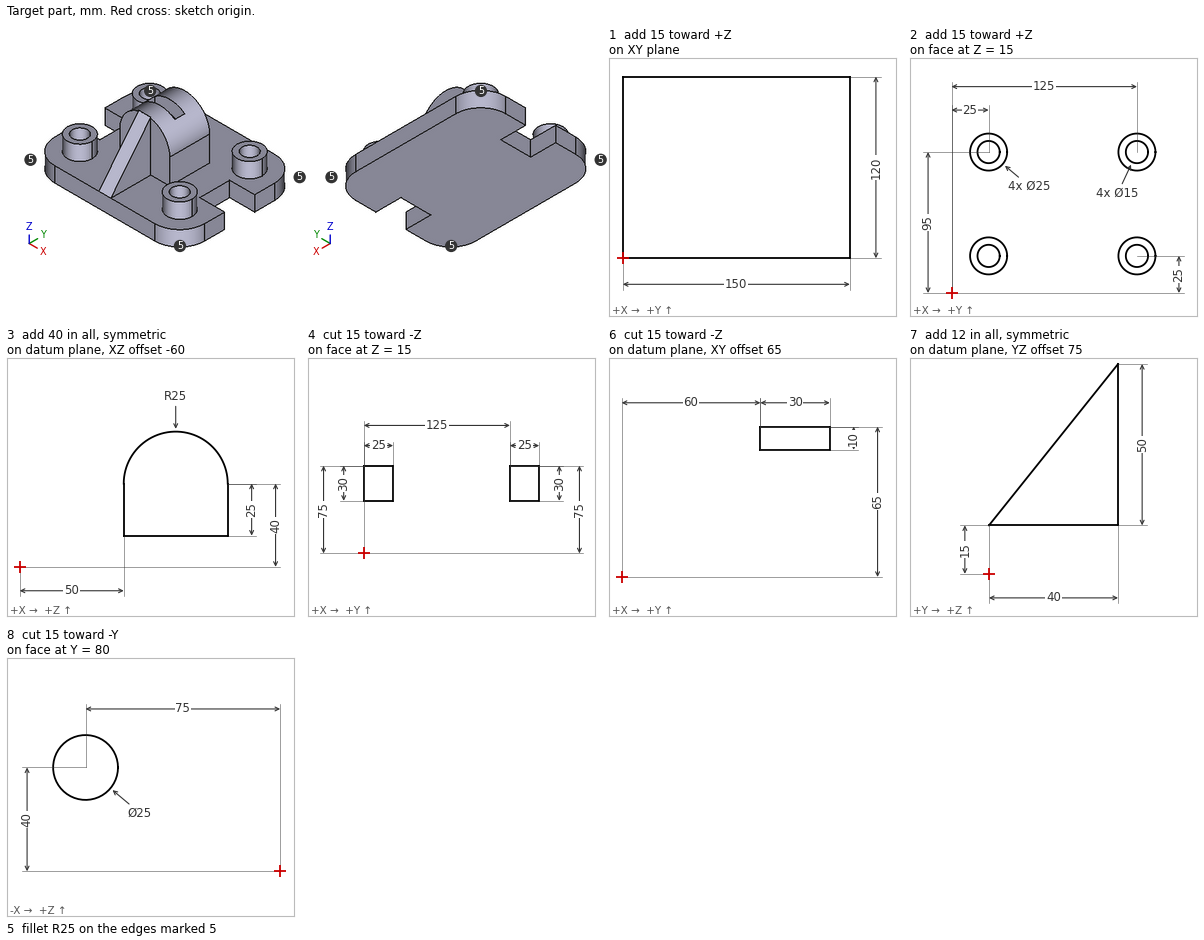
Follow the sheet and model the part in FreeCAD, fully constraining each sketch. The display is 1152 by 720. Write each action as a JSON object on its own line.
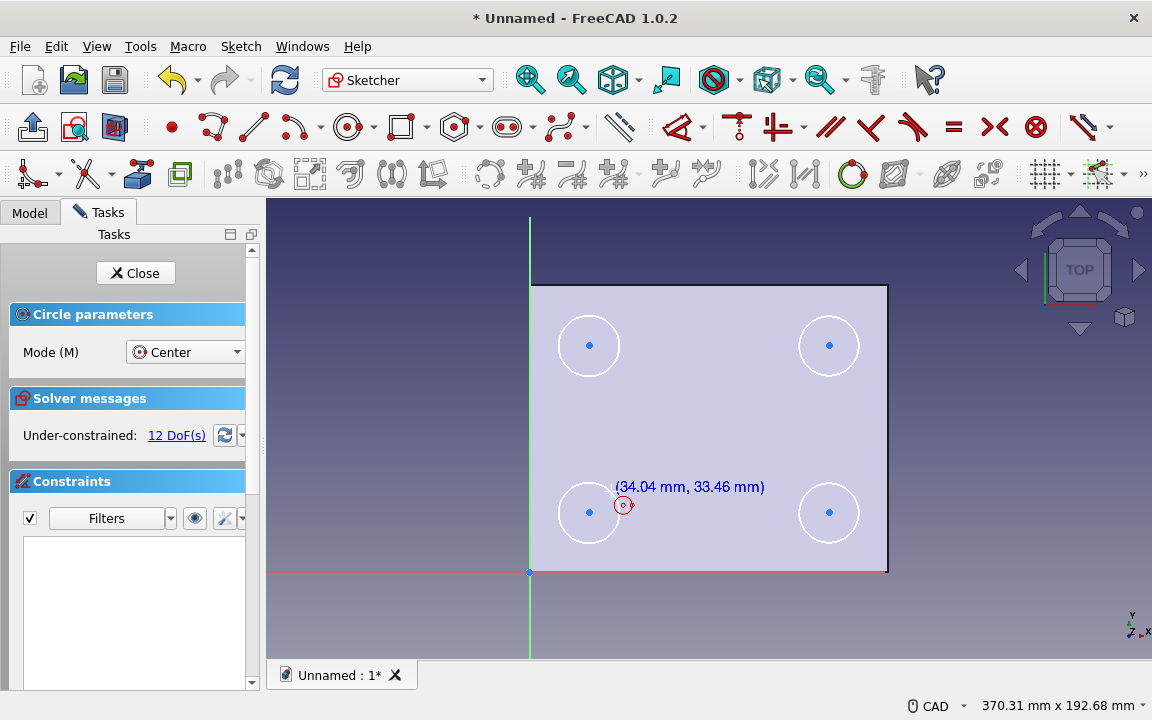
{"action": "scroll", "coordinate": [589, 345], "scroll_direction": "up", "scroll_amount": 2}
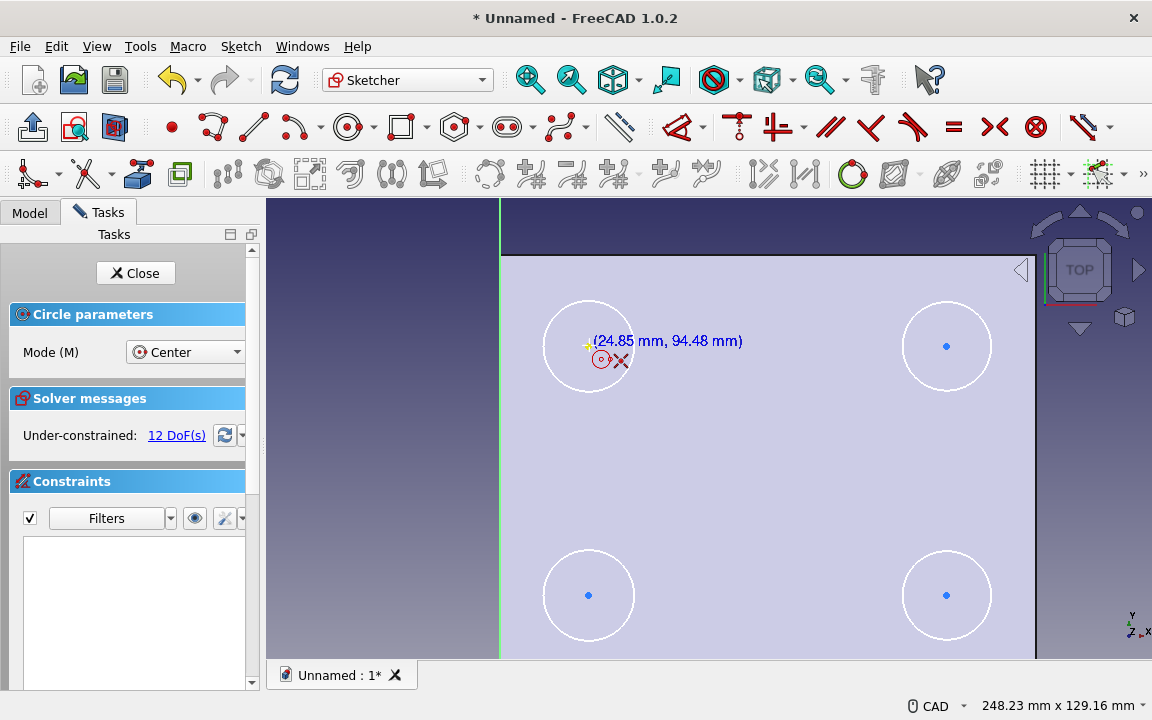
{"action": "left_click", "coordinate": [589, 346]}
{"action": "left_click", "coordinate": [608, 326]}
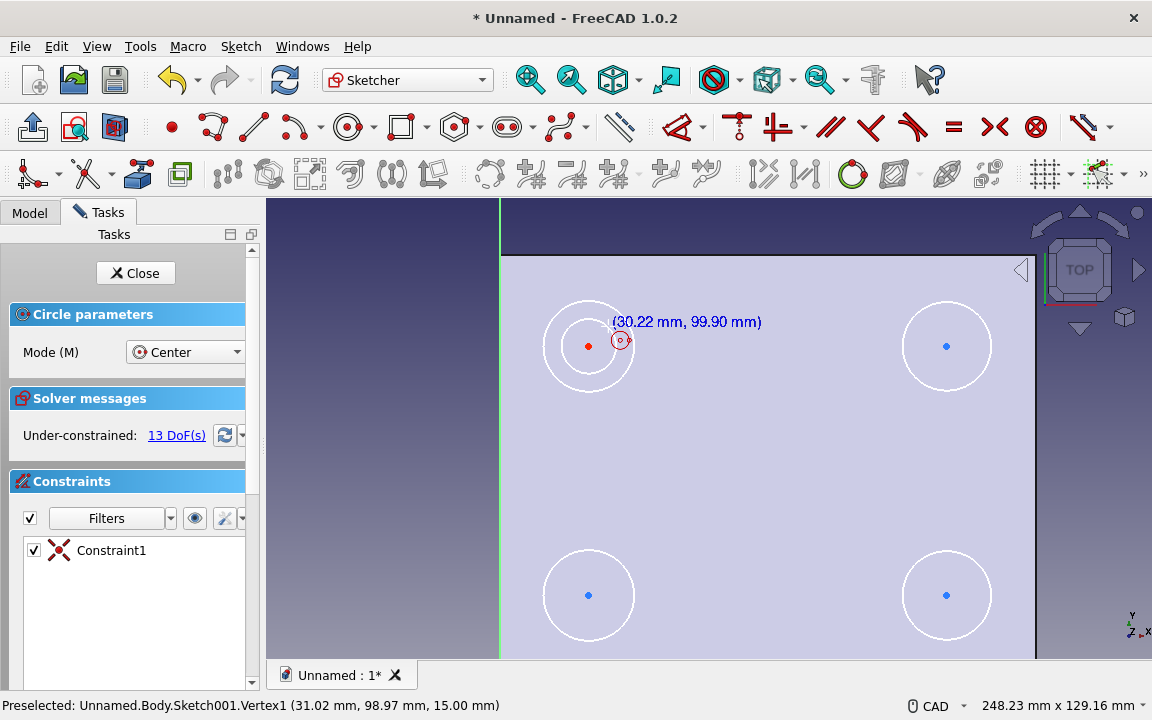
{"action": "left_click", "coordinate": [947, 346]}
{"action": "left_click", "coordinate": [965, 326]}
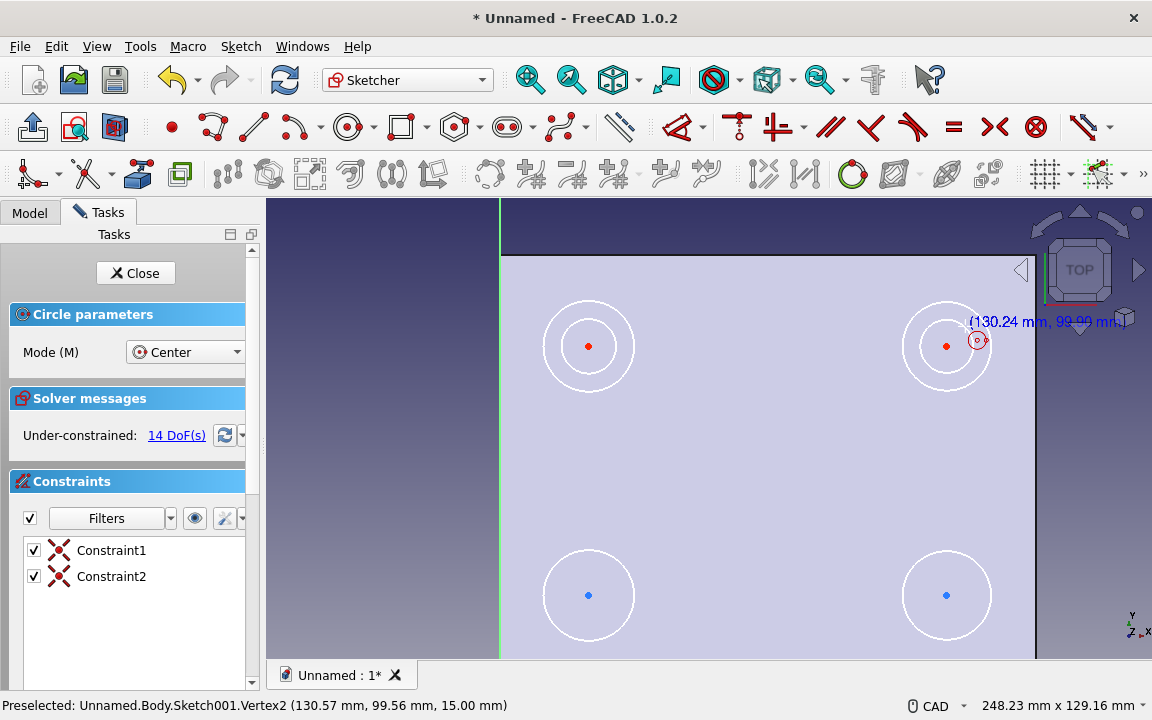
{"action": "left_click", "coordinate": [947, 595]}
{"action": "left_click", "coordinate": [965, 575]}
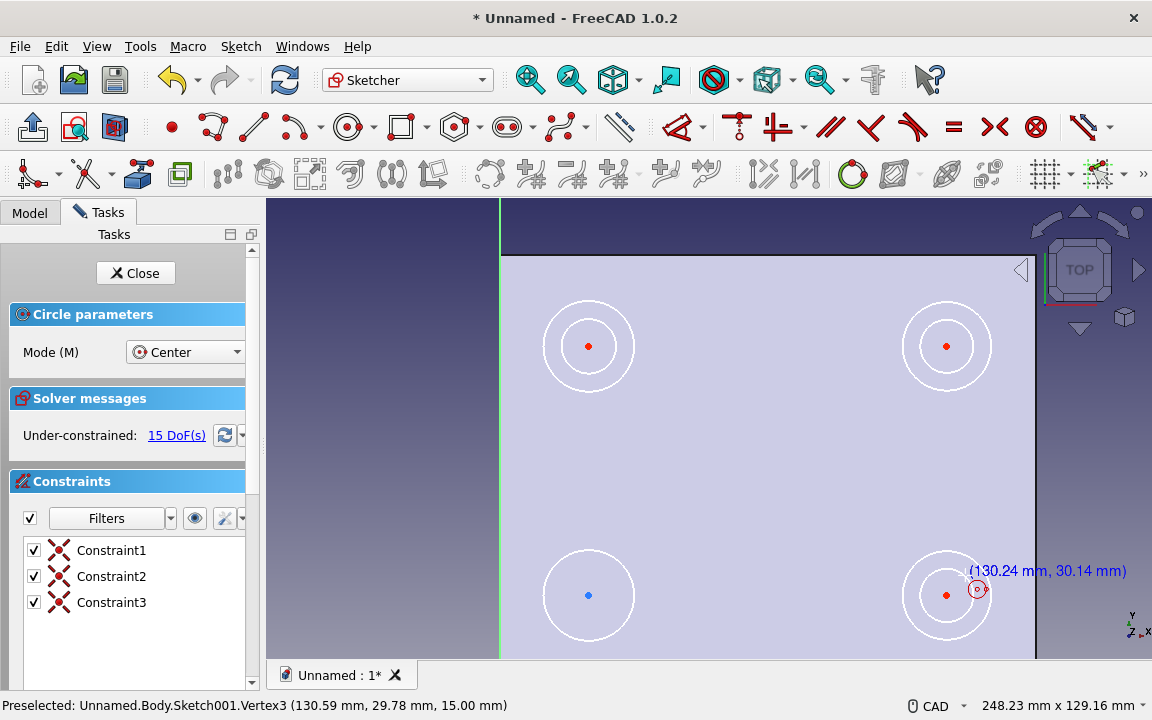
{"action": "left_click", "coordinate": [589, 595]}
{"action": "left_click", "coordinate": [608, 575]}
{"action": "key", "text": "Escape"}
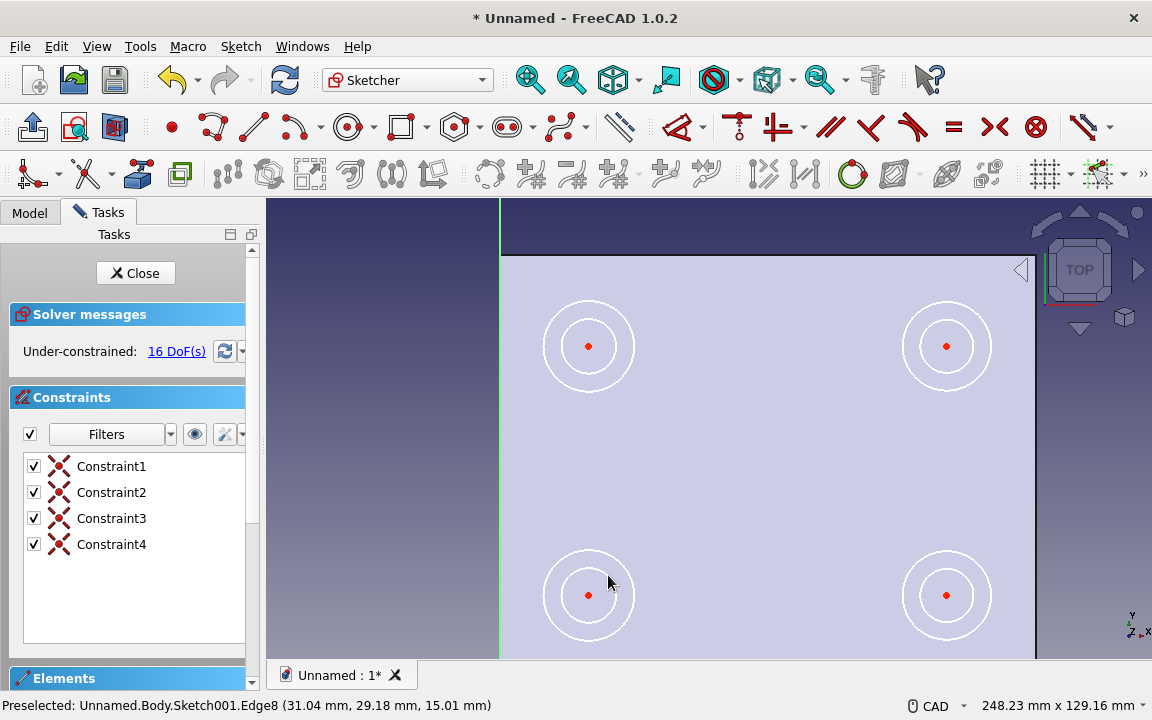
{"action": "left_click", "coordinate": [621, 314]}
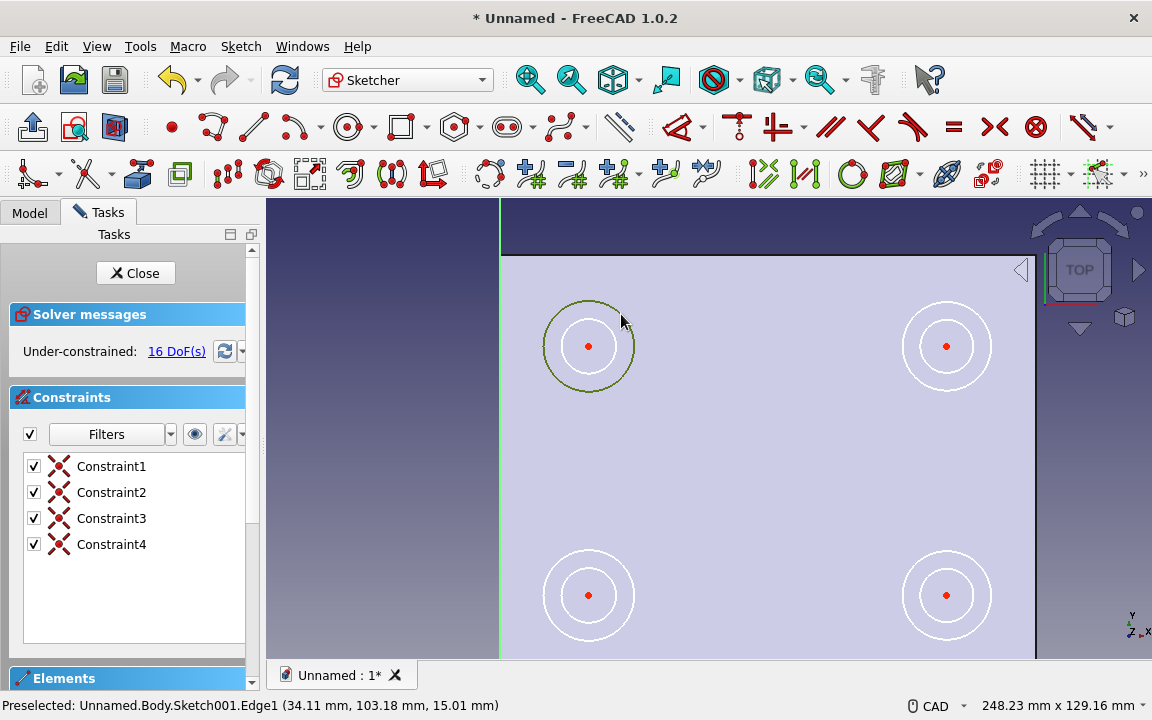
{"action": "left_click", "coordinate": [978, 315]}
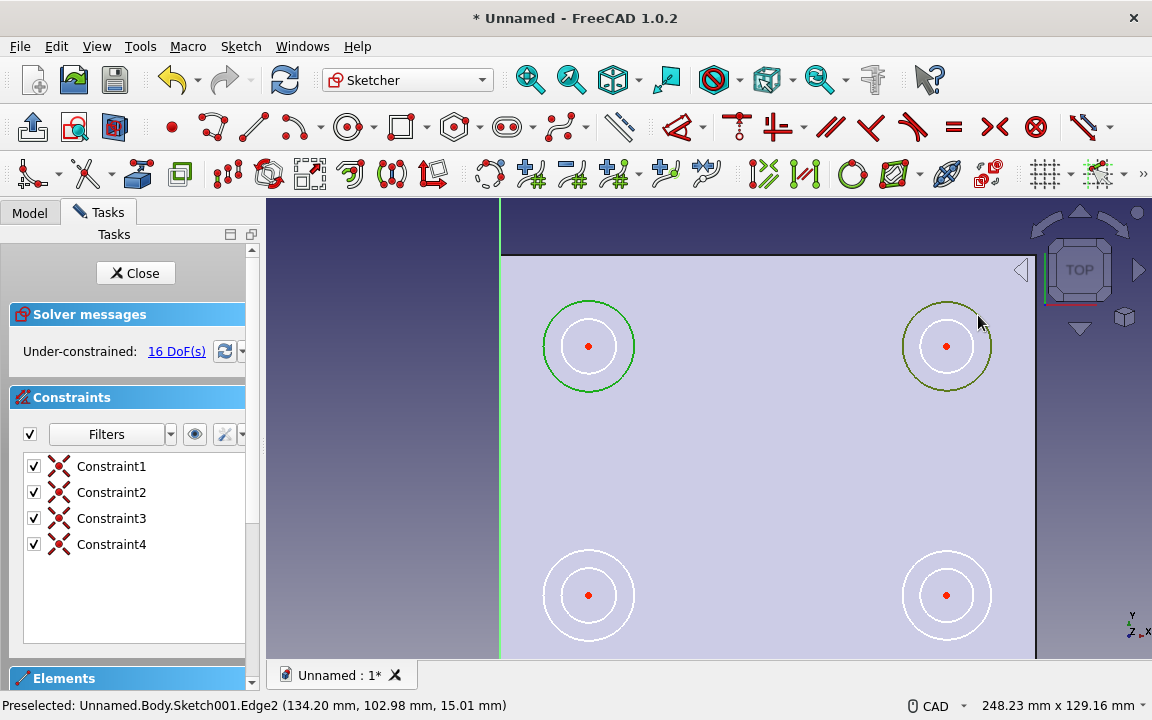
{"action": "left_click", "coordinate": [978, 564]}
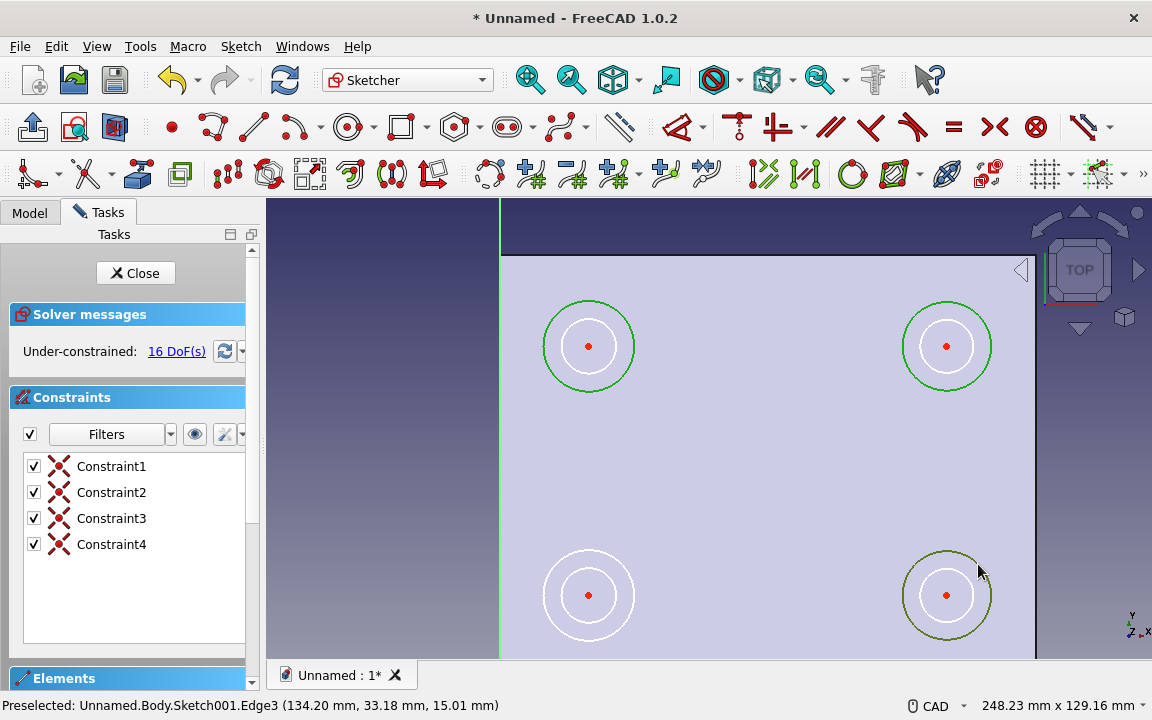
{"action": "left_click", "coordinate": [621, 563]}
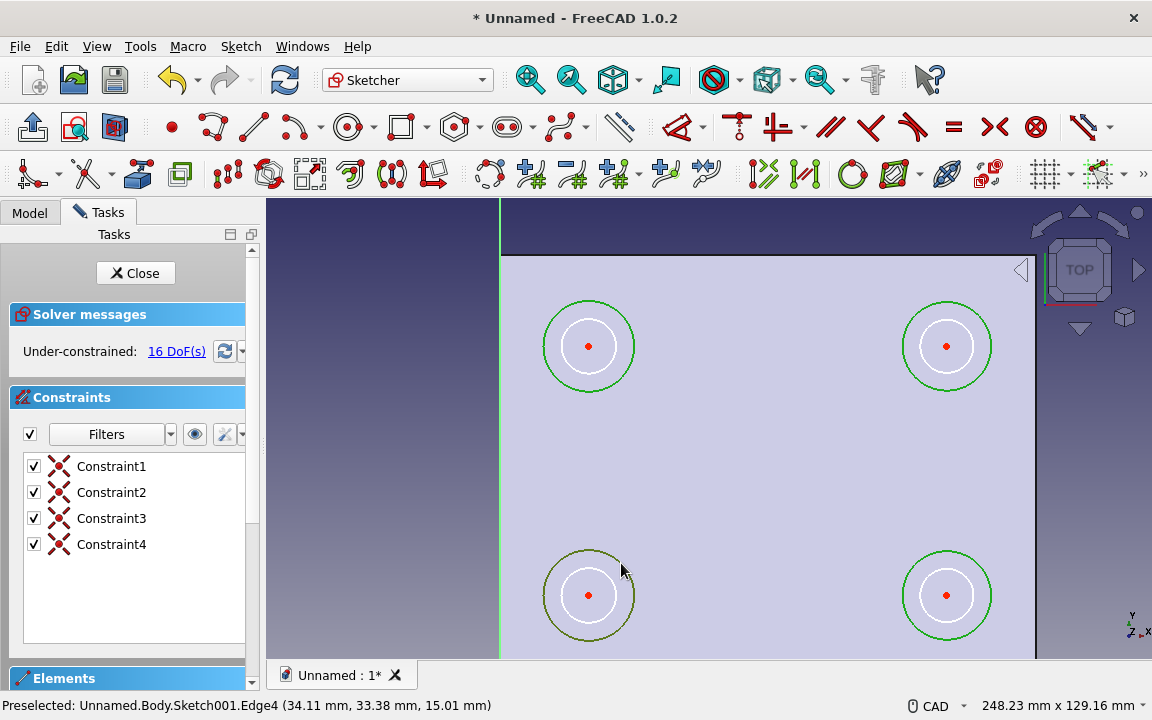
{"action": "left_click", "coordinate": [954, 128]}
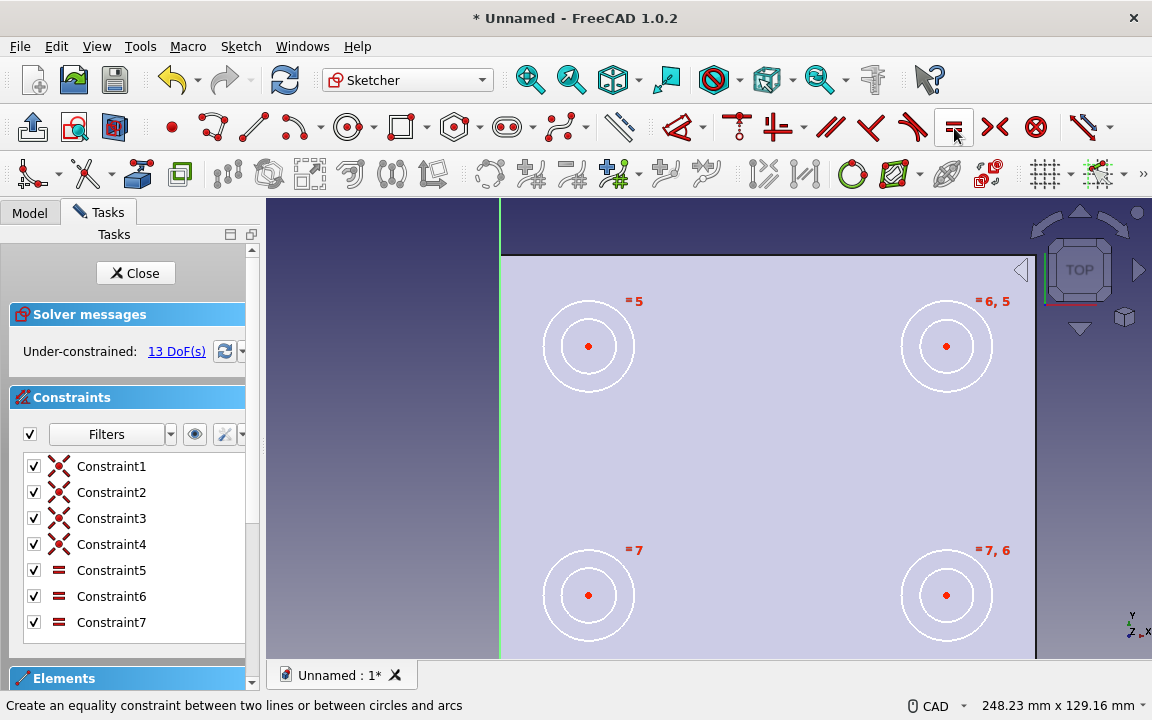
{"action": "left_click", "coordinate": [608, 327]}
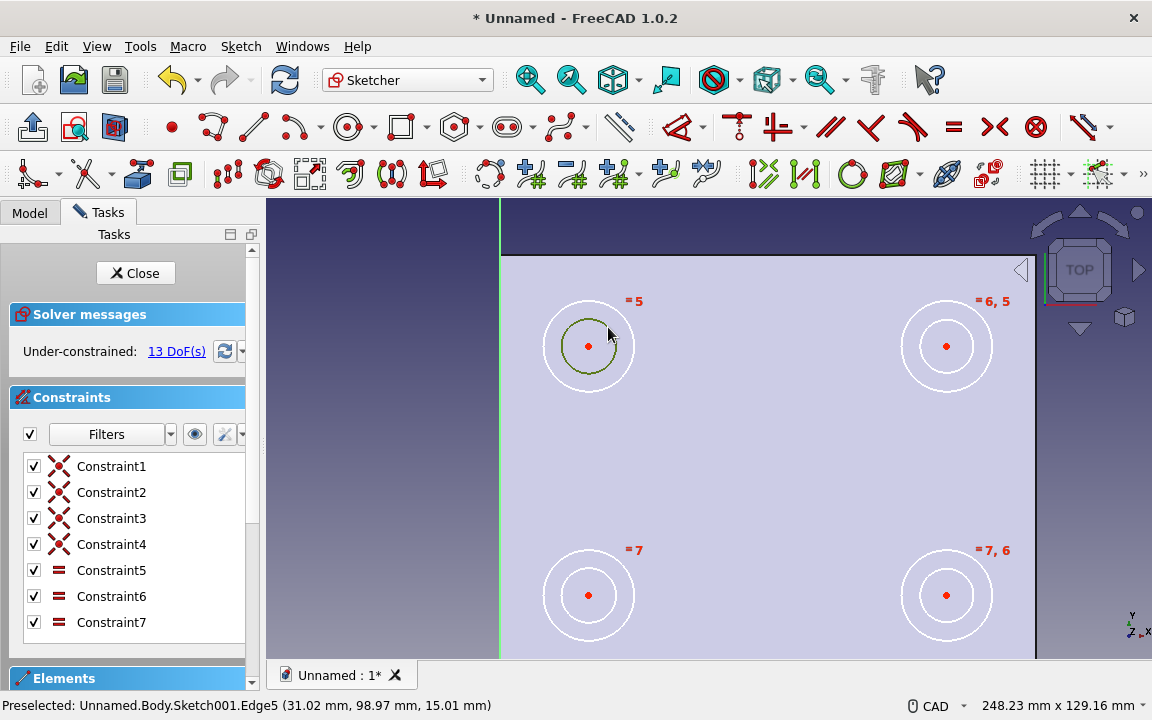
{"action": "left_click", "coordinate": [966, 328]}